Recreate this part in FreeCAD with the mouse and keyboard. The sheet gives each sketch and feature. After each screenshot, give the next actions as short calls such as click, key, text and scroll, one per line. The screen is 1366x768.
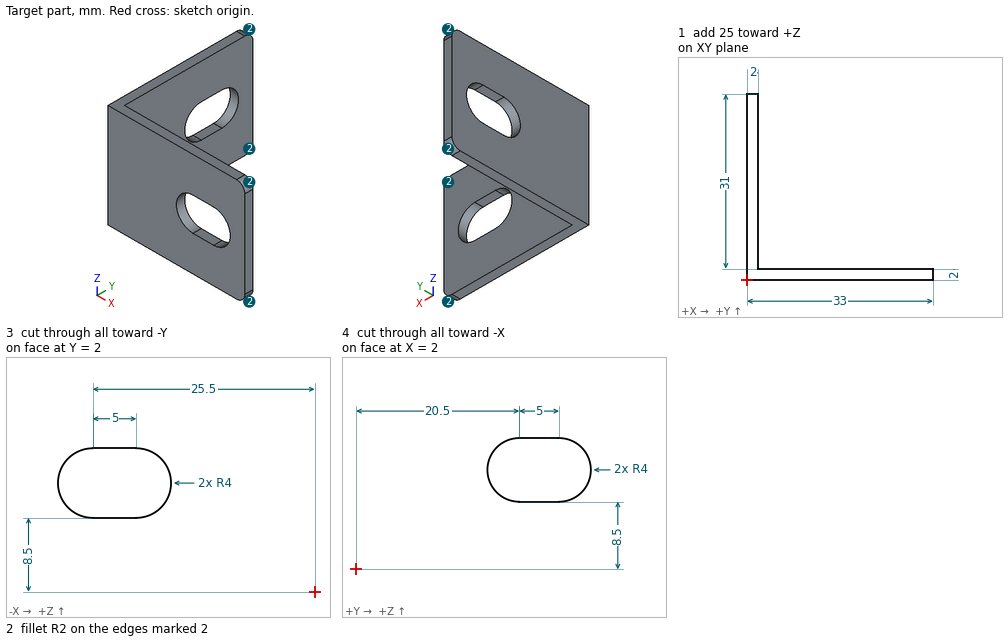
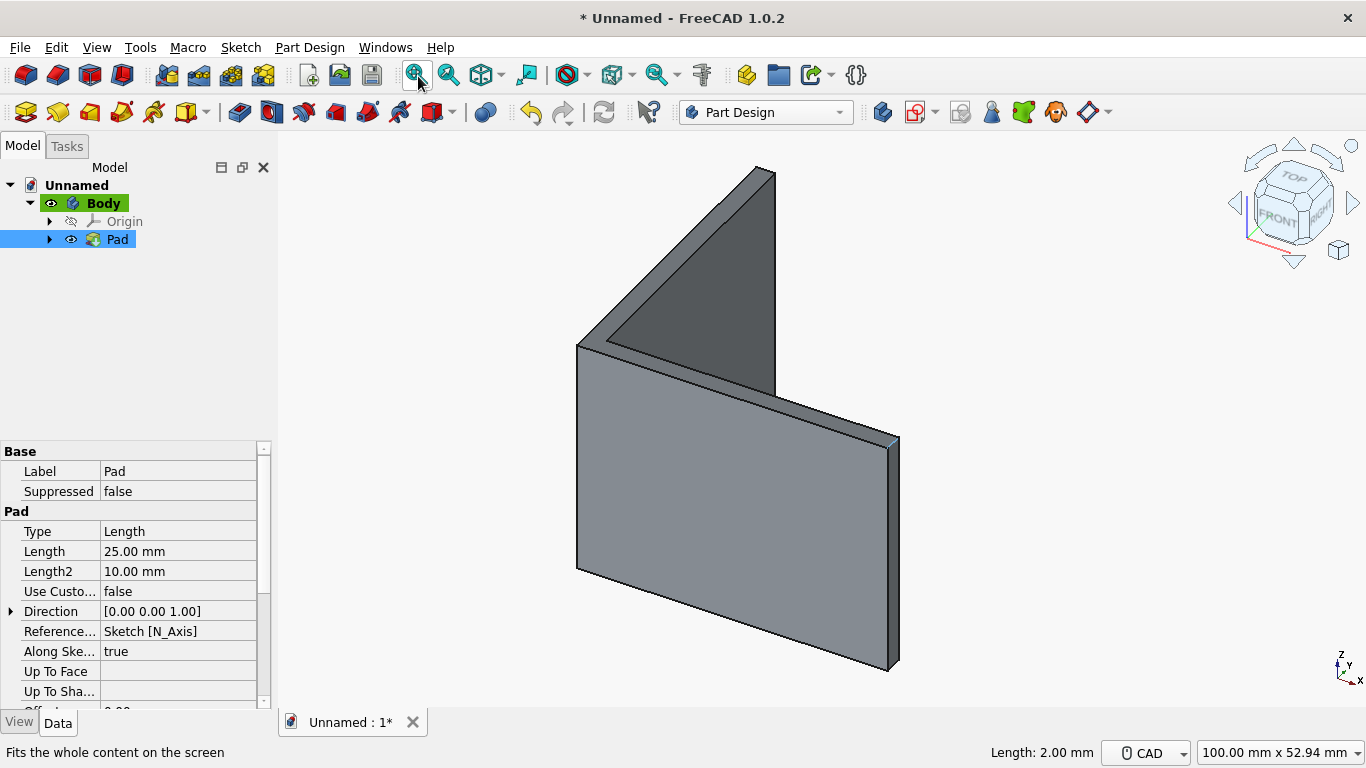
key(0)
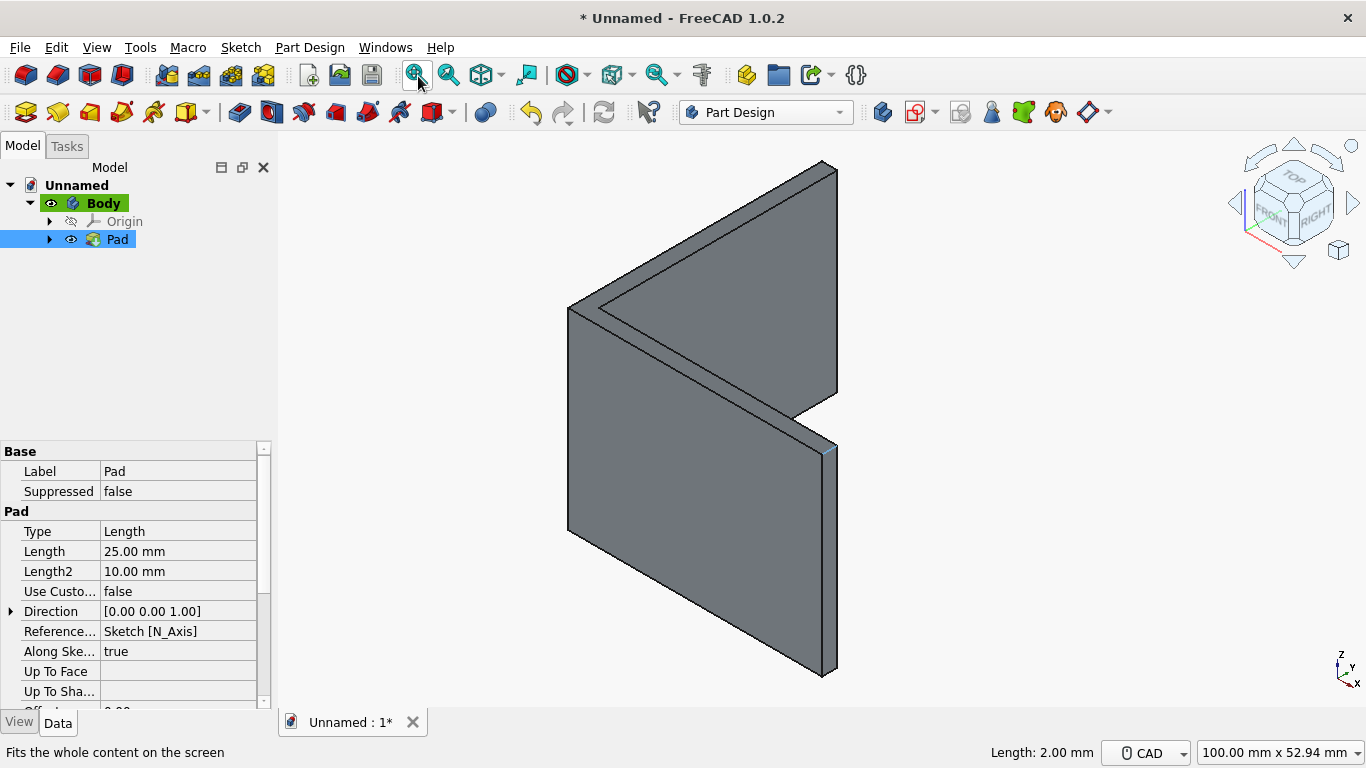
scroll(830, 165, up, 4)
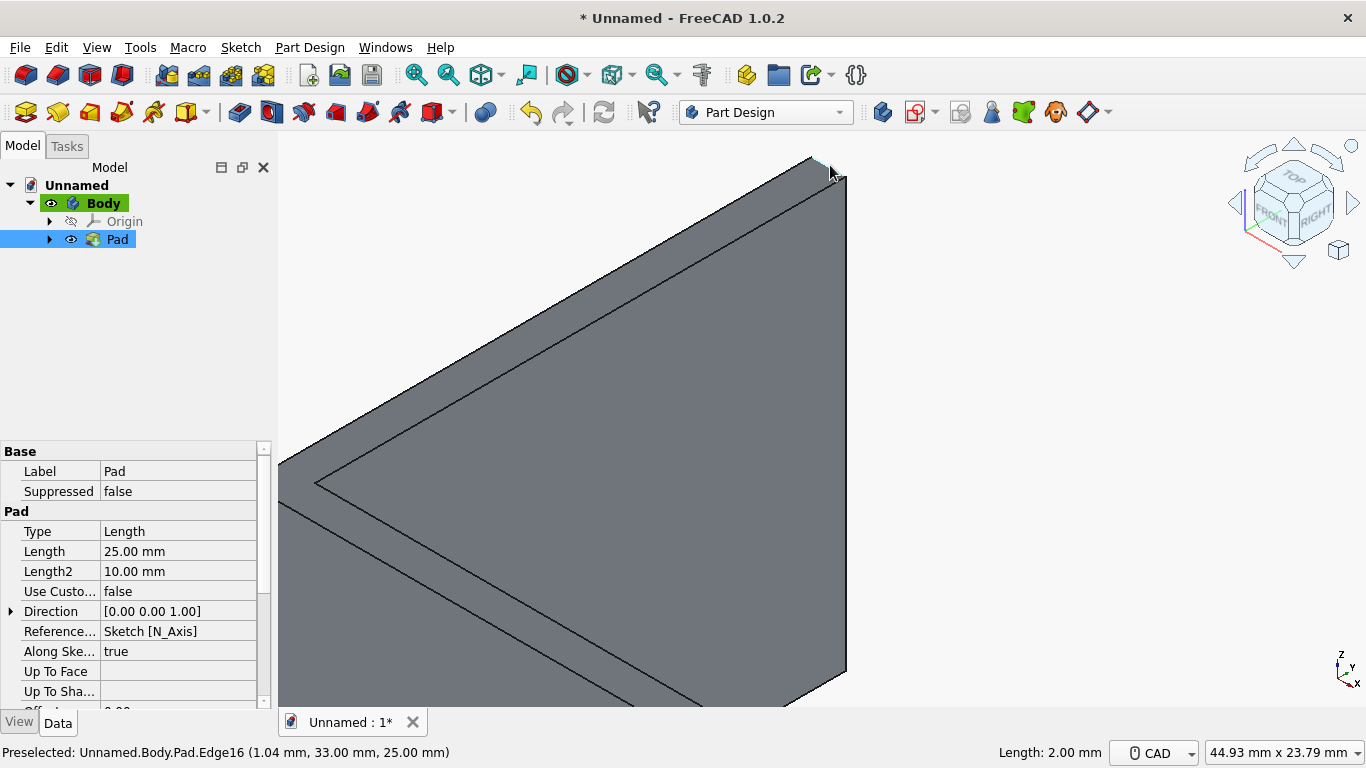
key(v)
key(f)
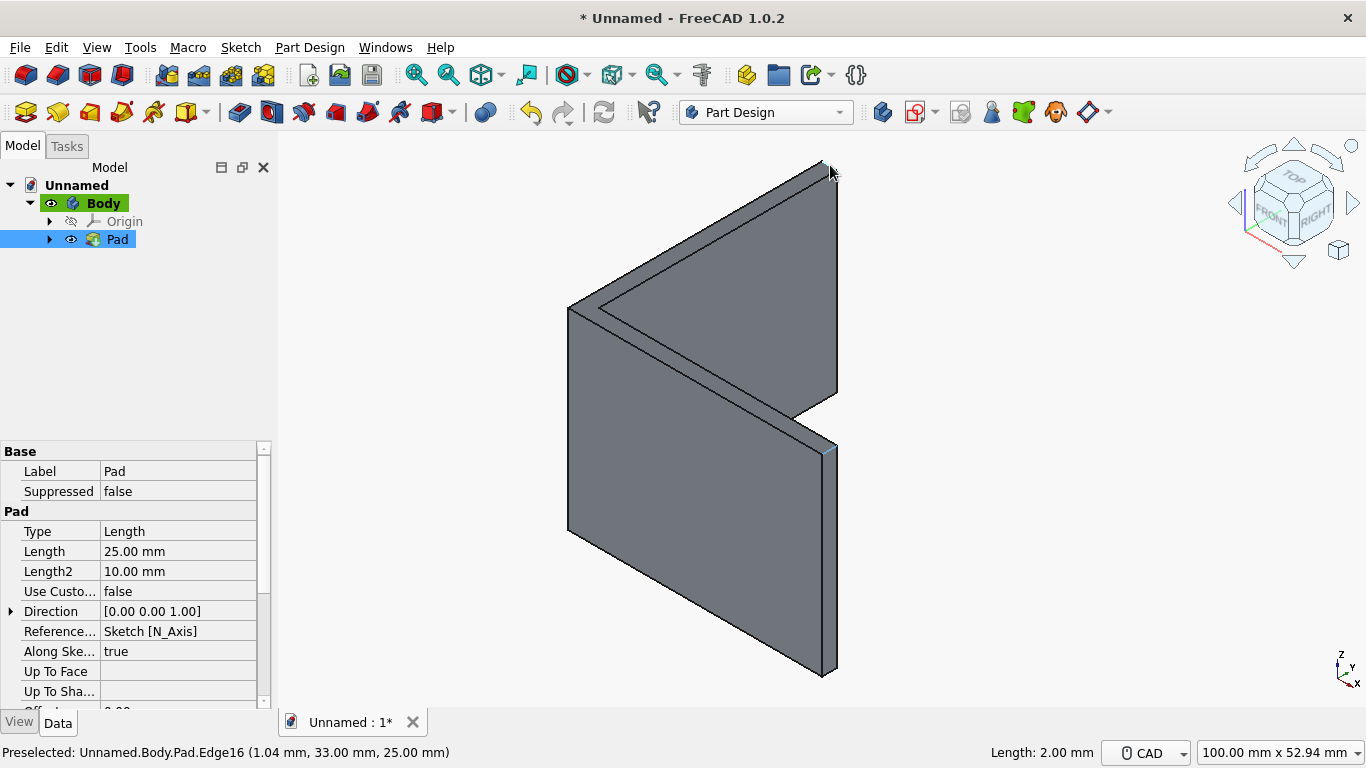
key(2)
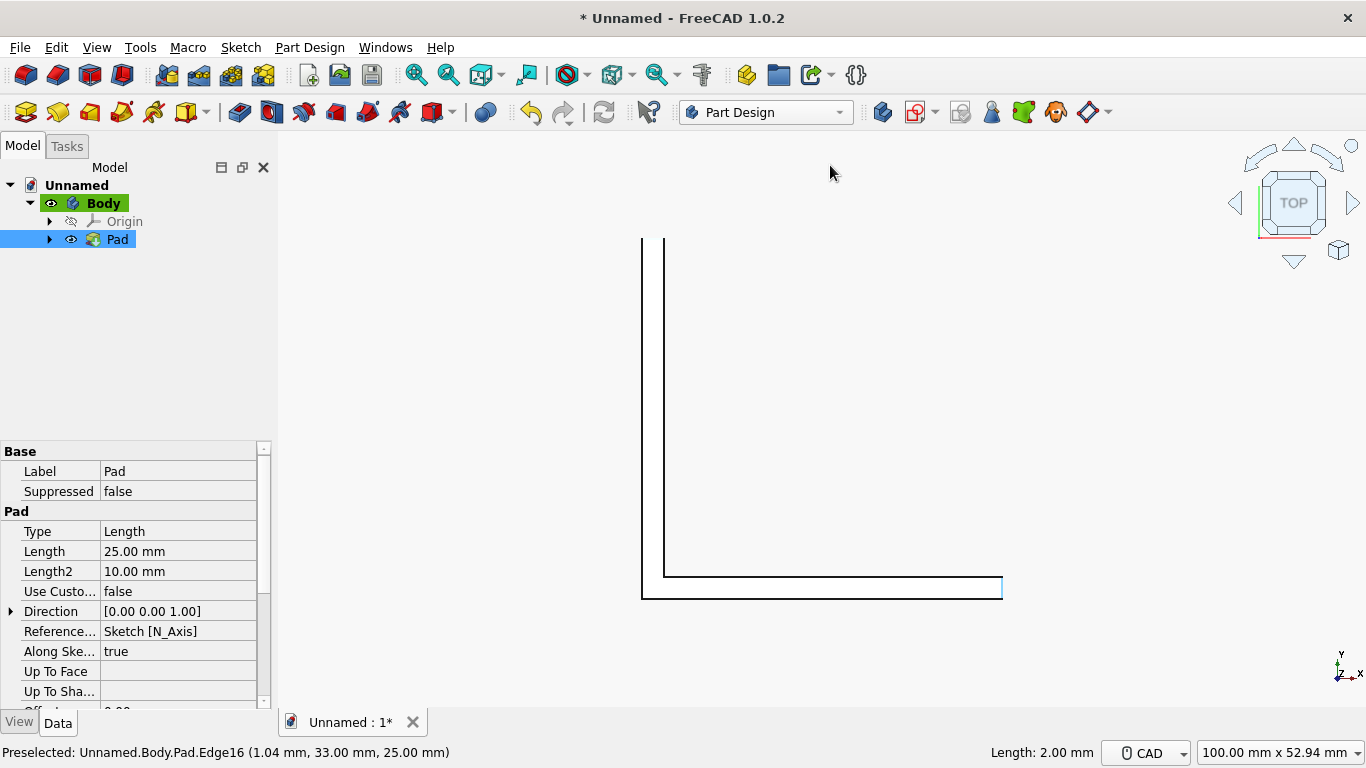
click(653, 238, ctrl)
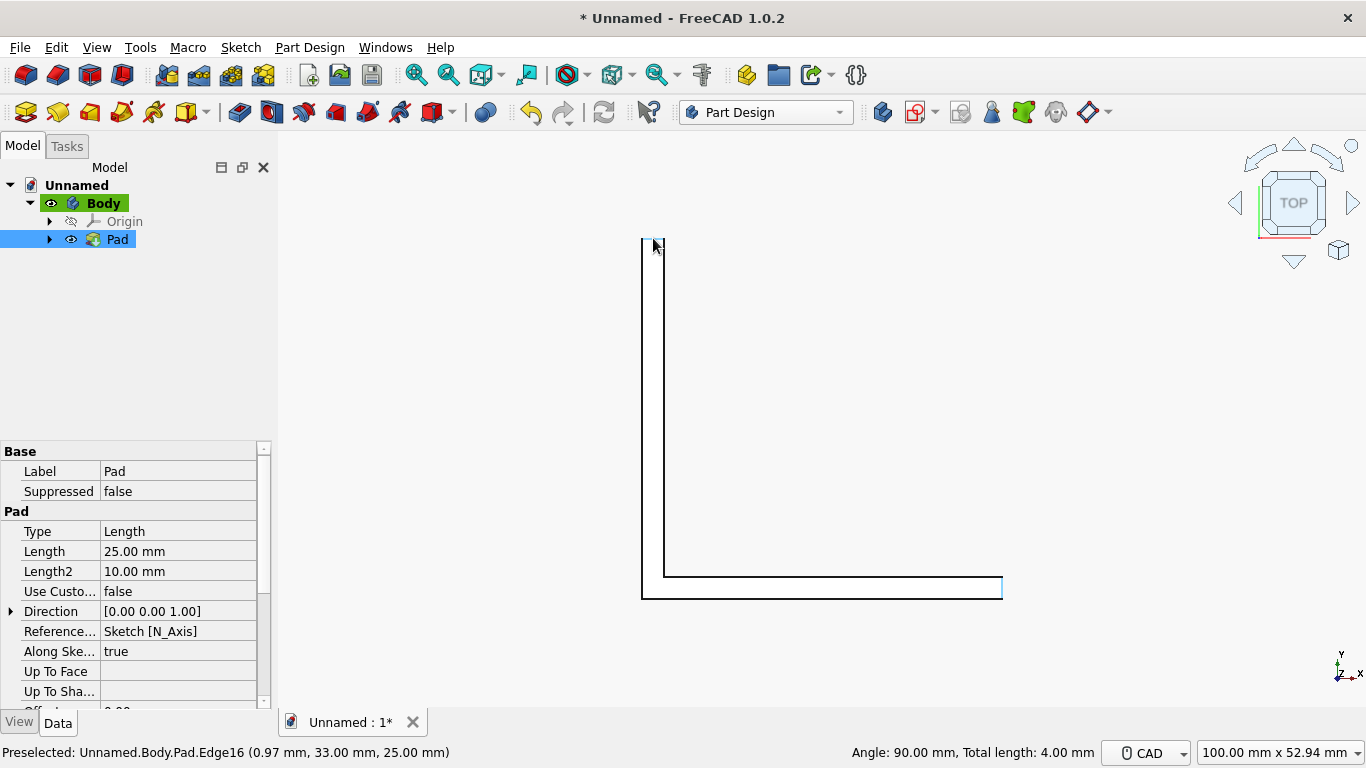
scroll(653, 238, up, 4)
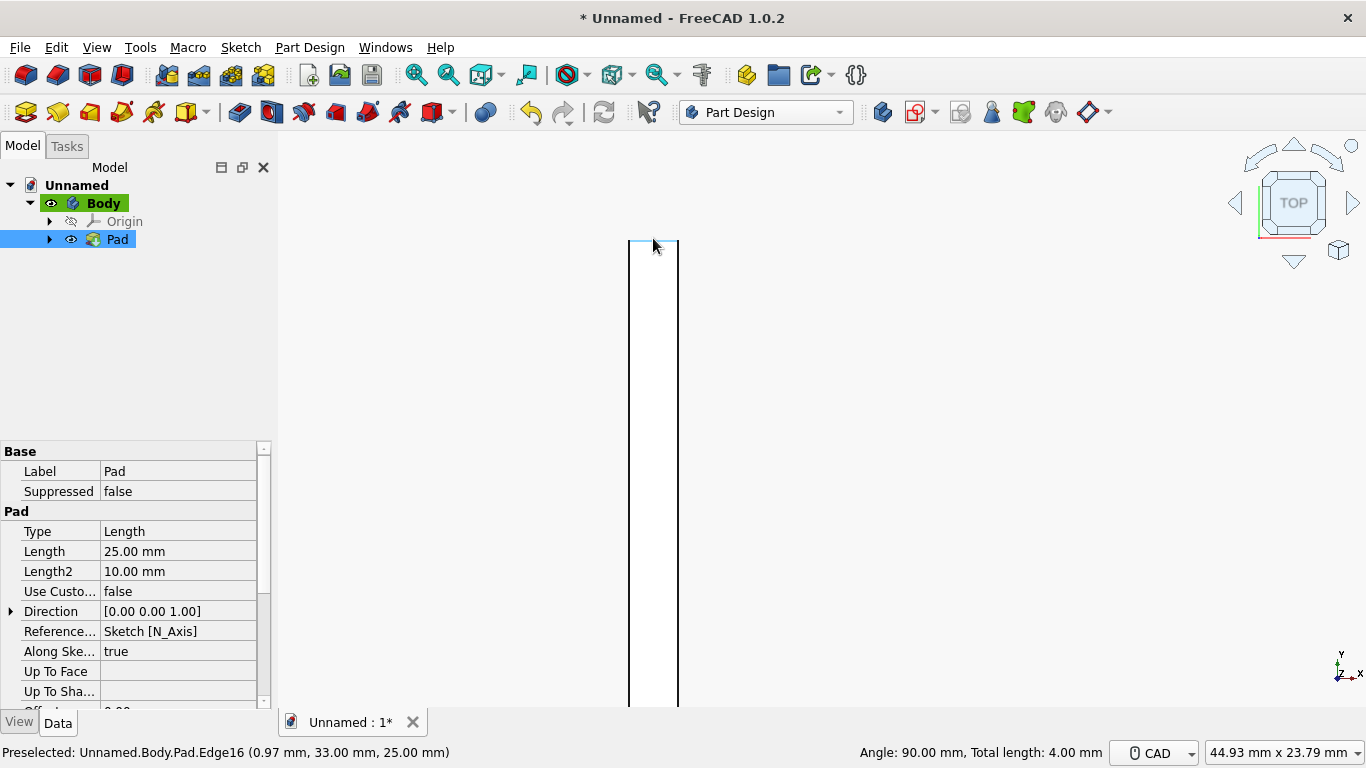
key(v)
key(f)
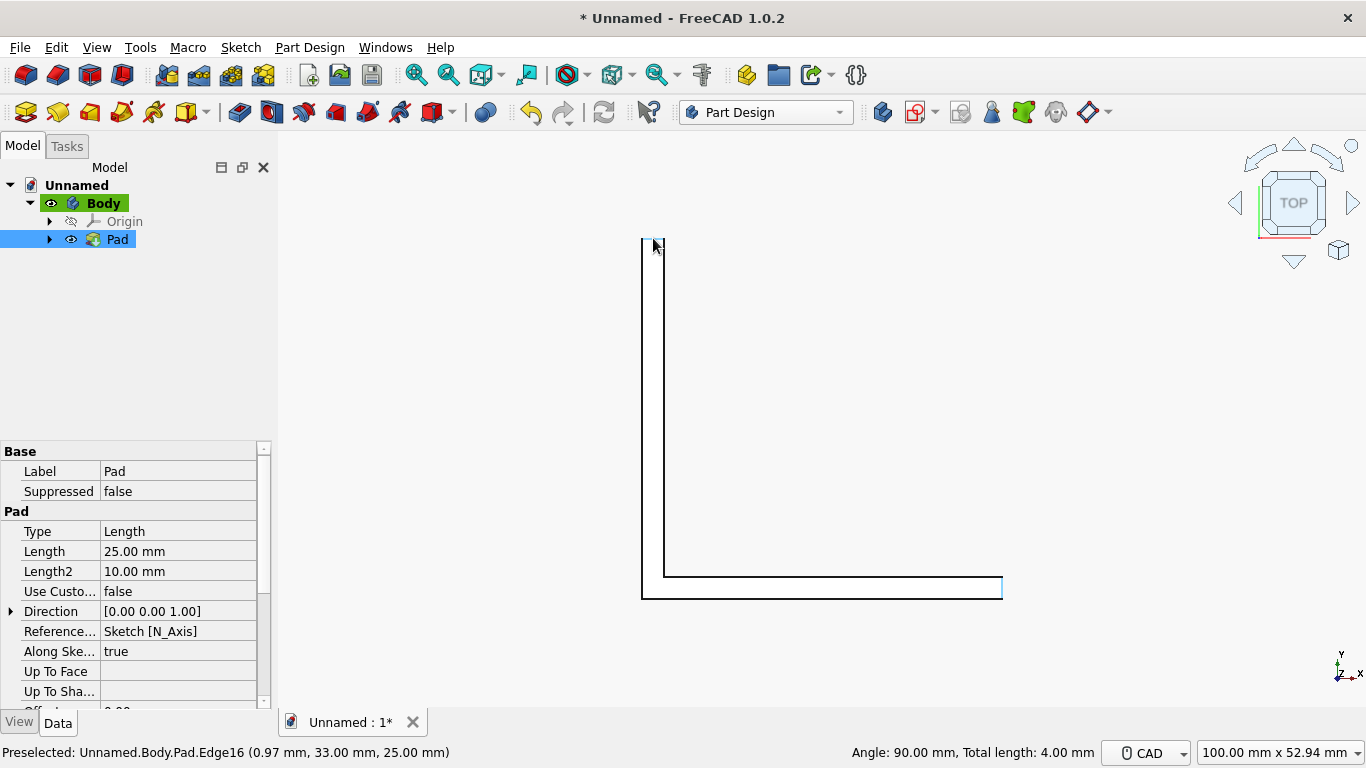
key(1)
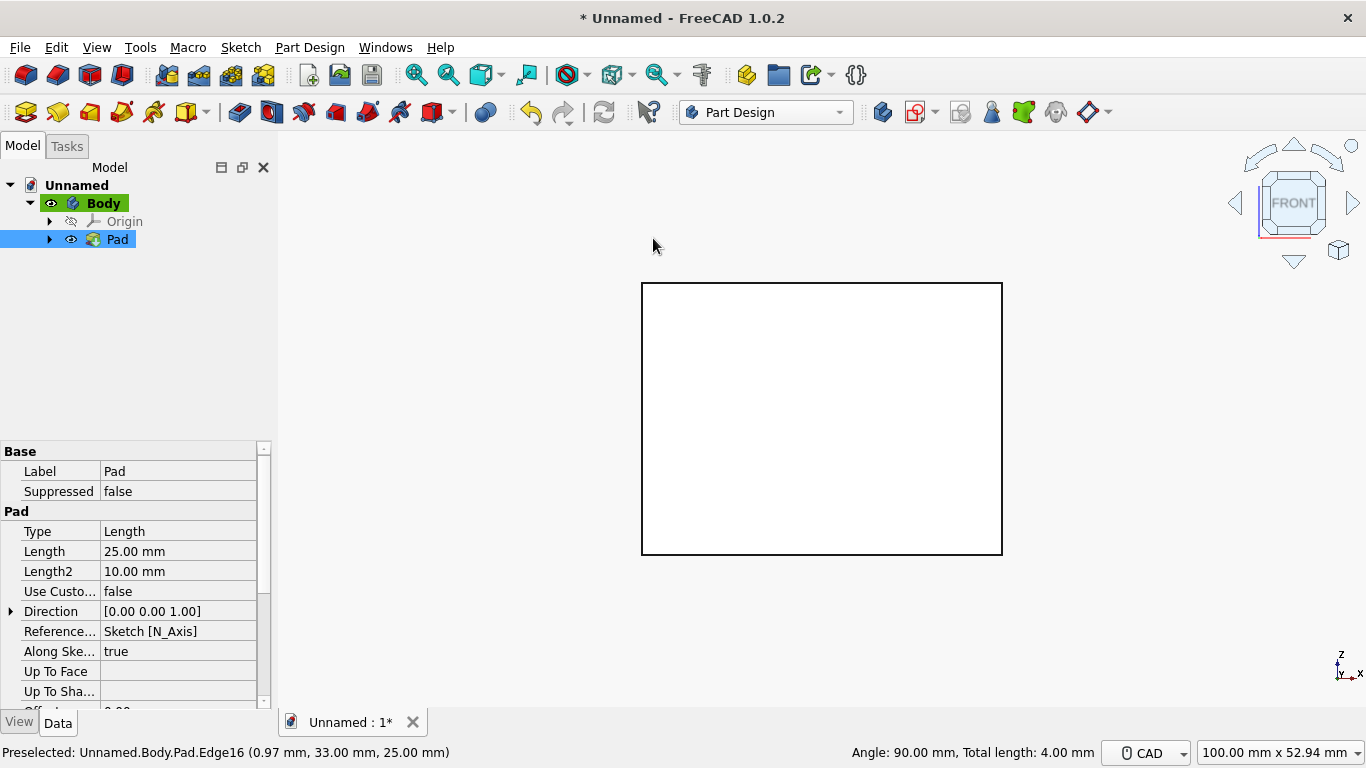
scroll(653, 554, up, 4)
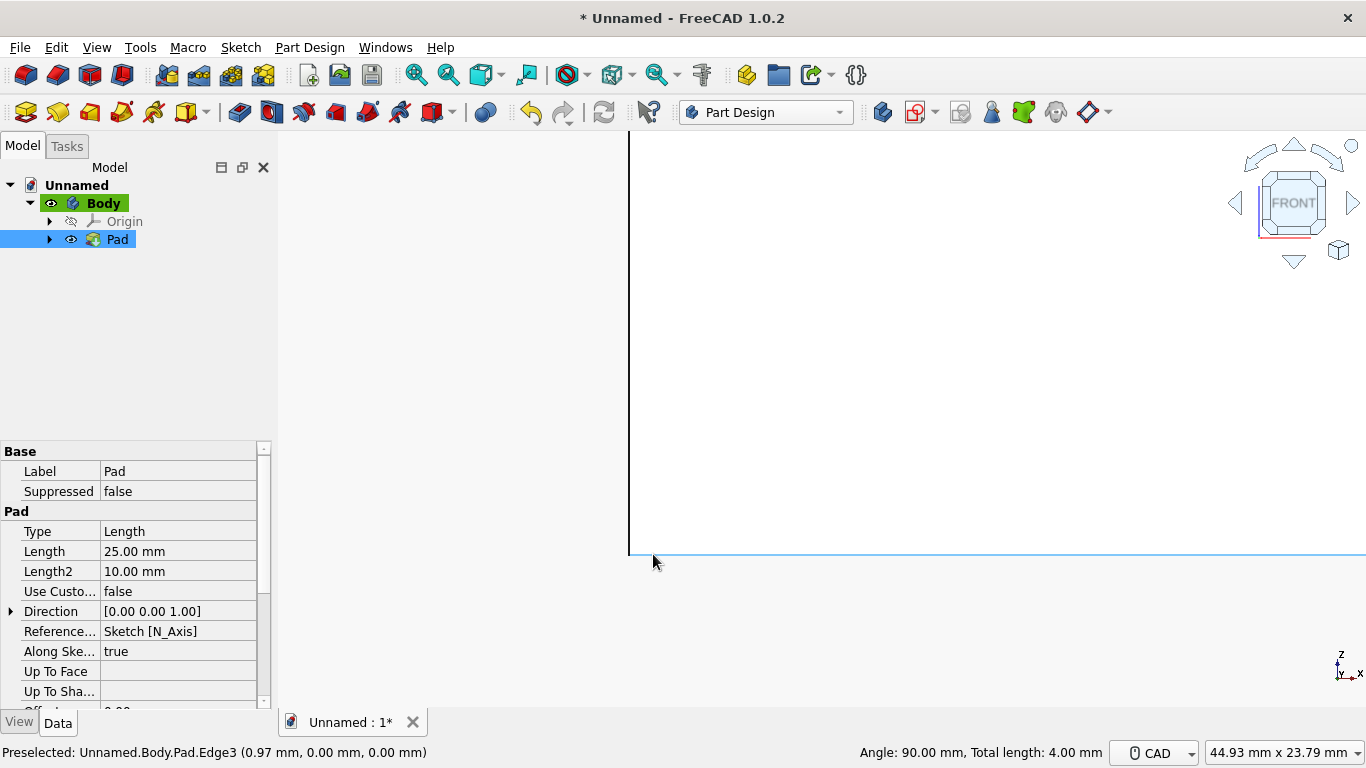
click(418, 76)